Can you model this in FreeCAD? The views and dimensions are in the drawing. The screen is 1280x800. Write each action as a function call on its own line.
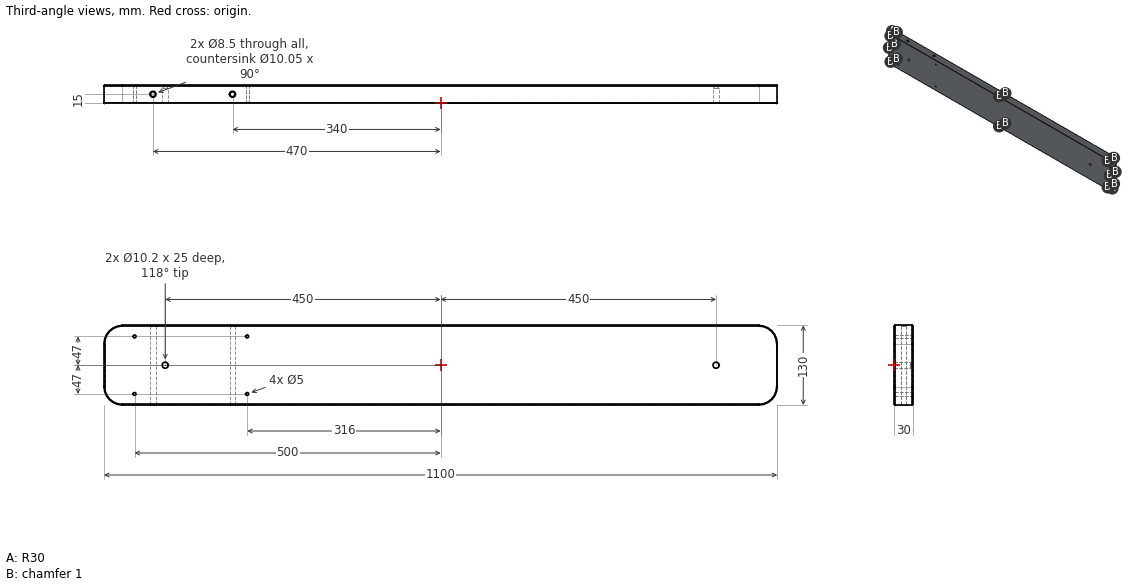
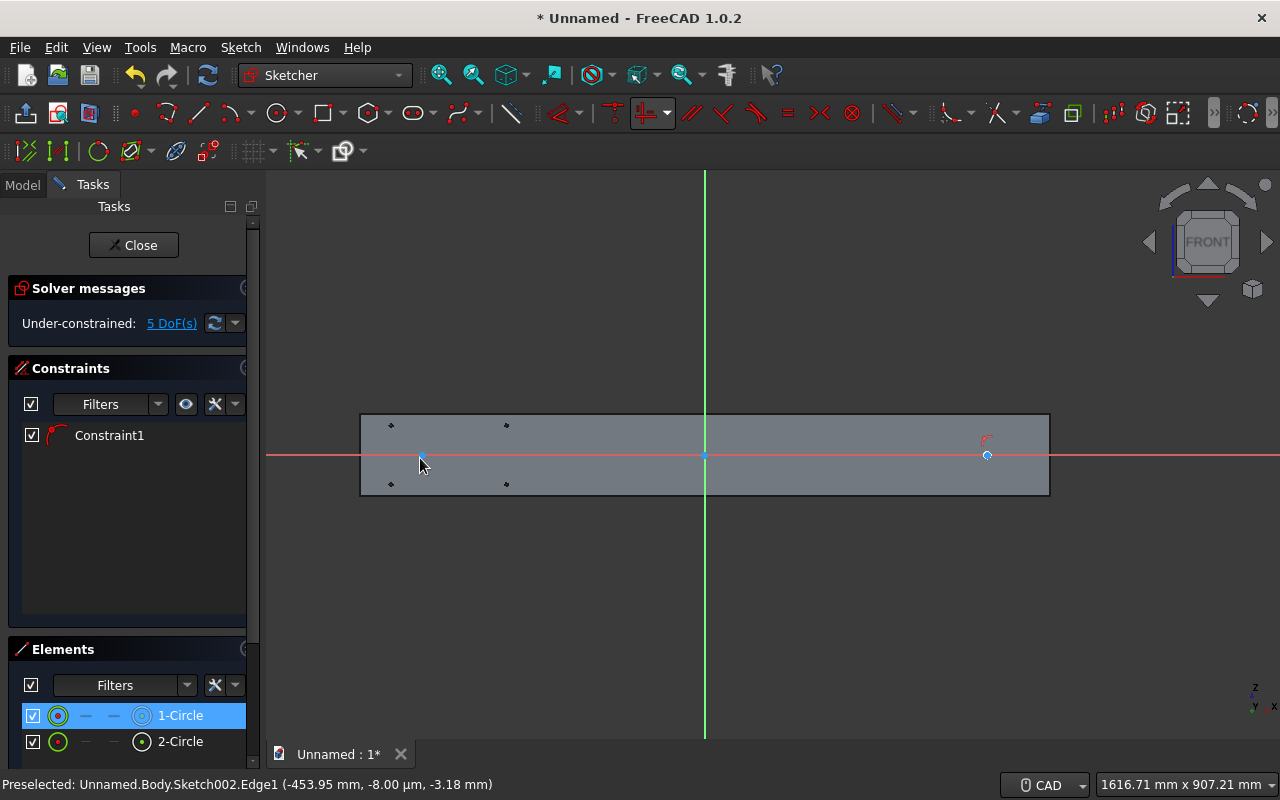
scroll(990, 453, up, 9)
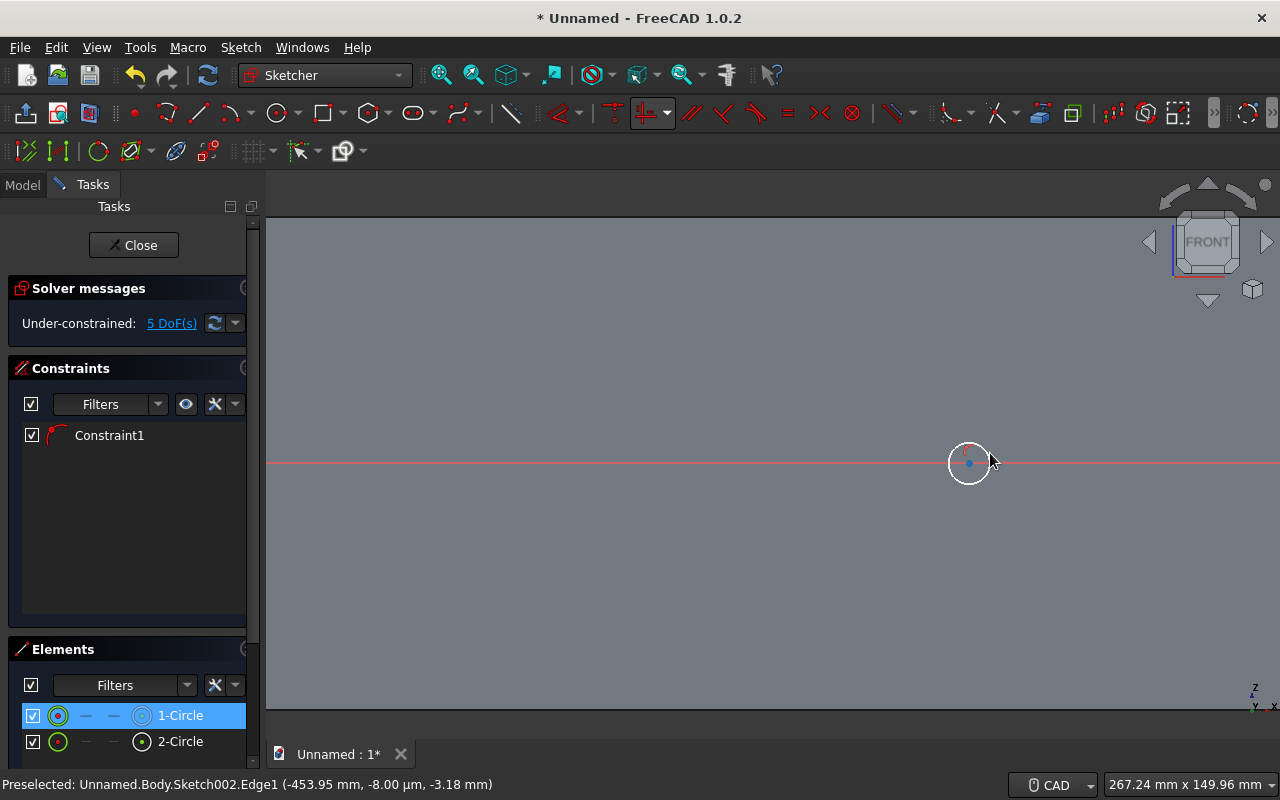
click(984, 449)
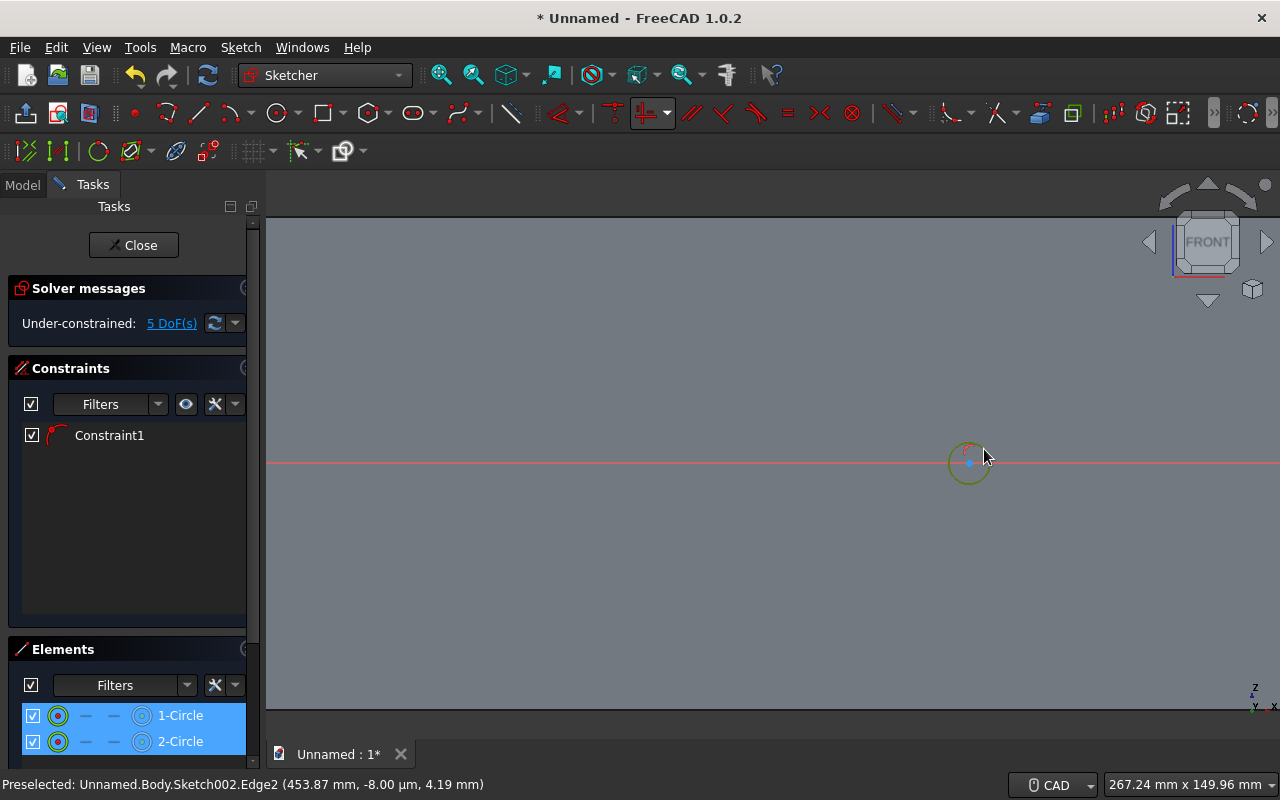
click(788, 114)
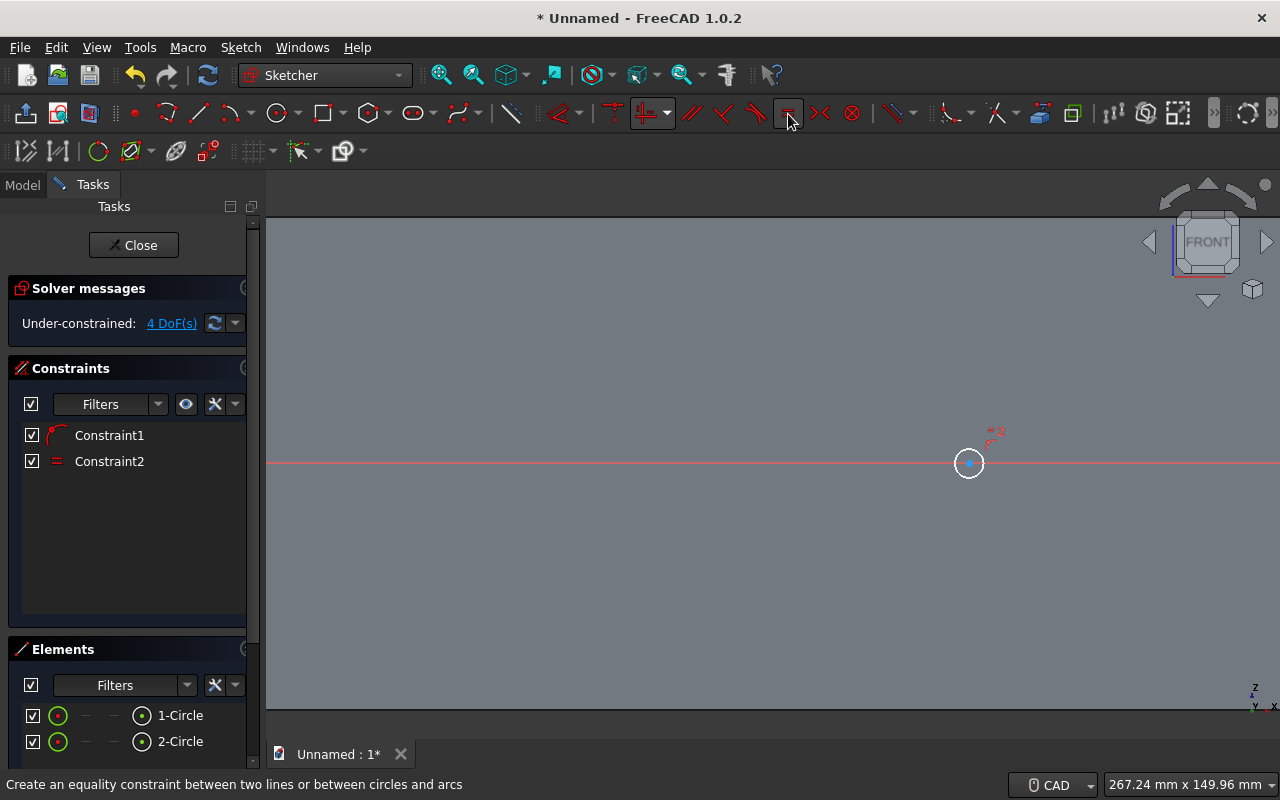
scroll(991, 453, down, 9)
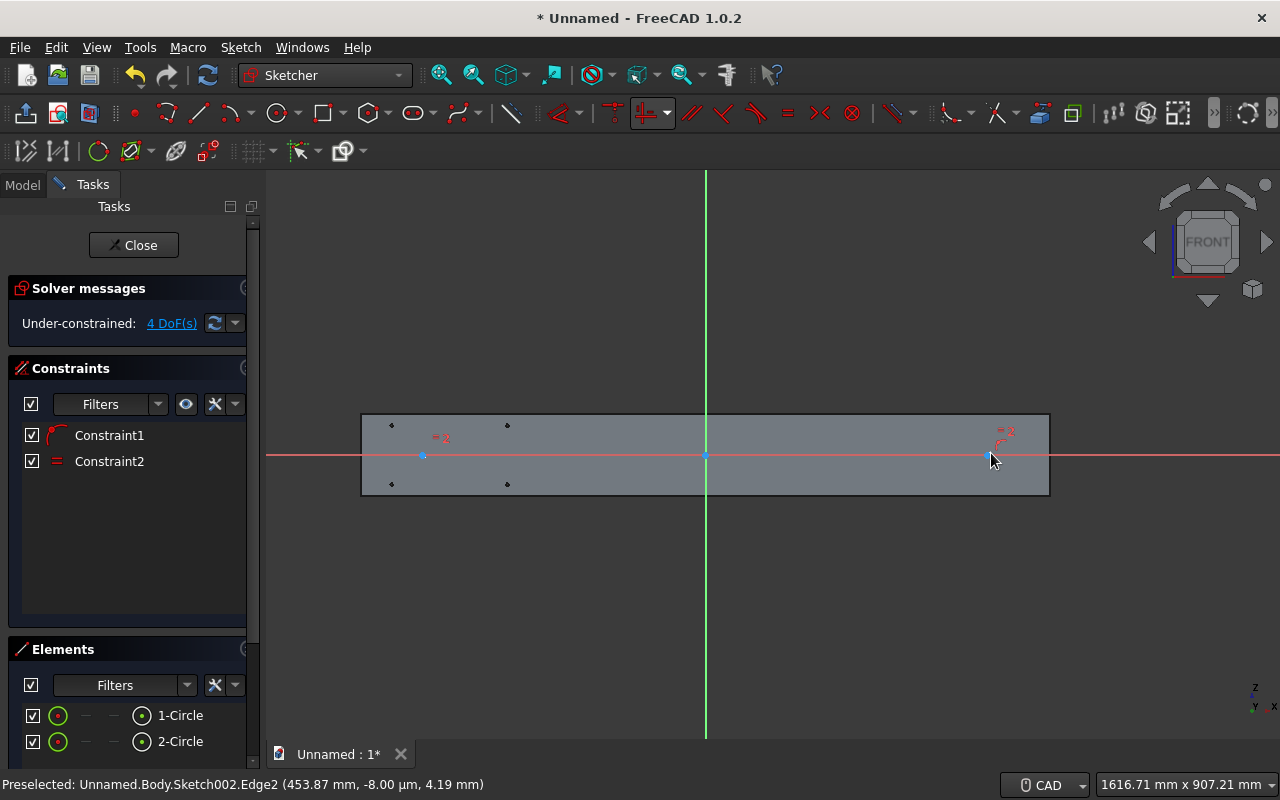
click(423, 456)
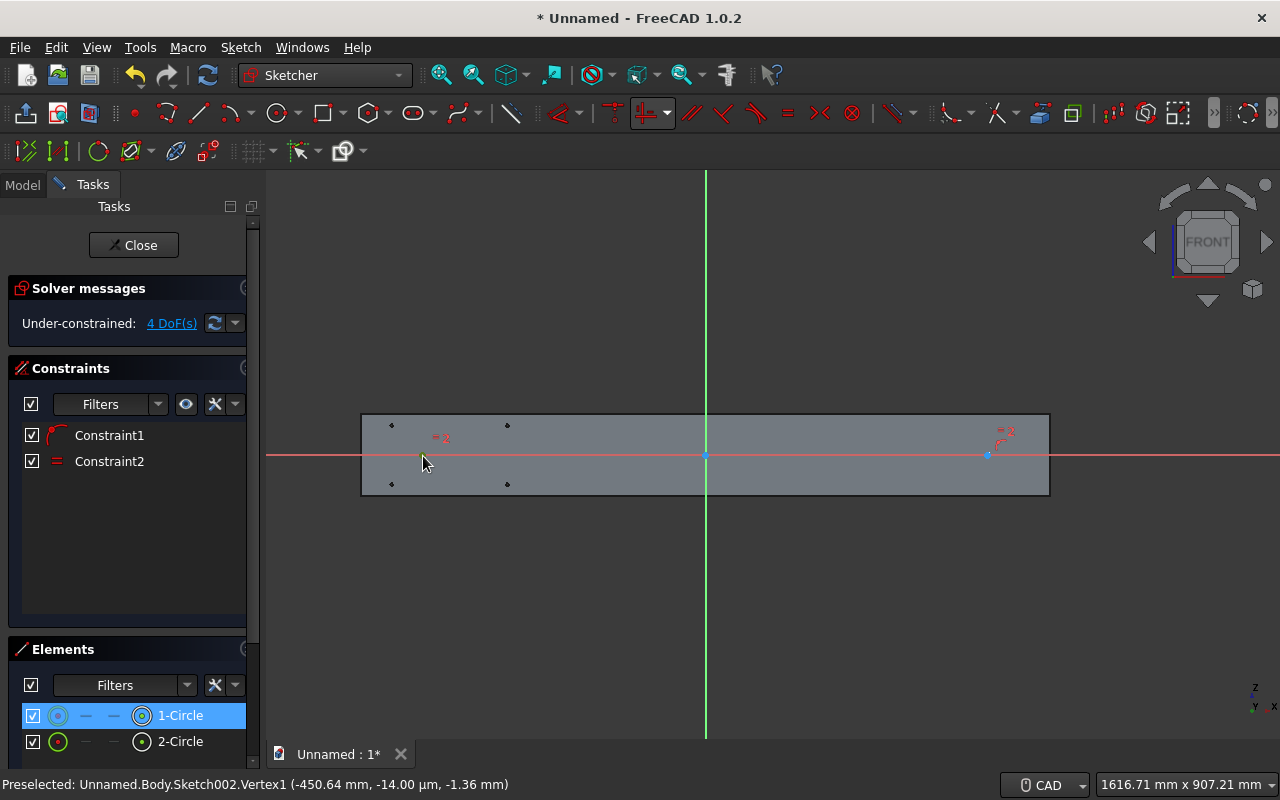
click(353, 455)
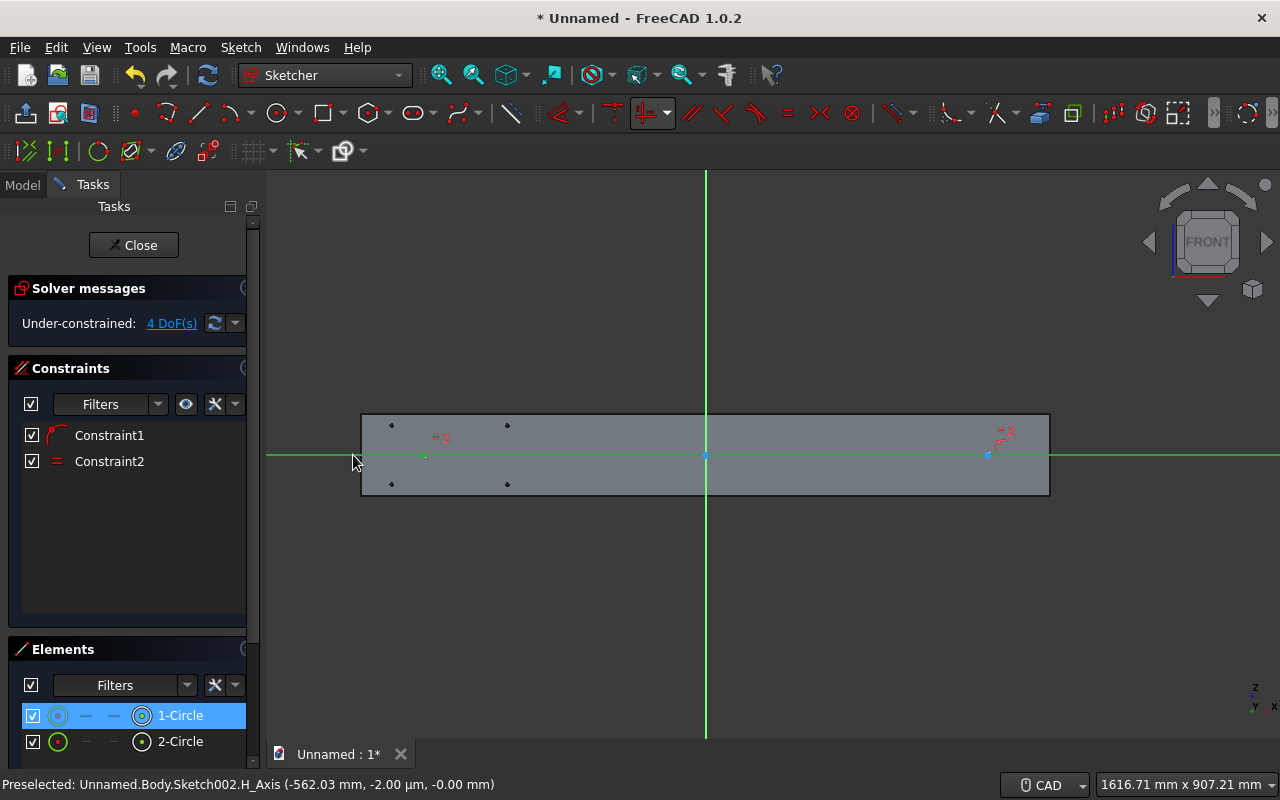
click(614, 114)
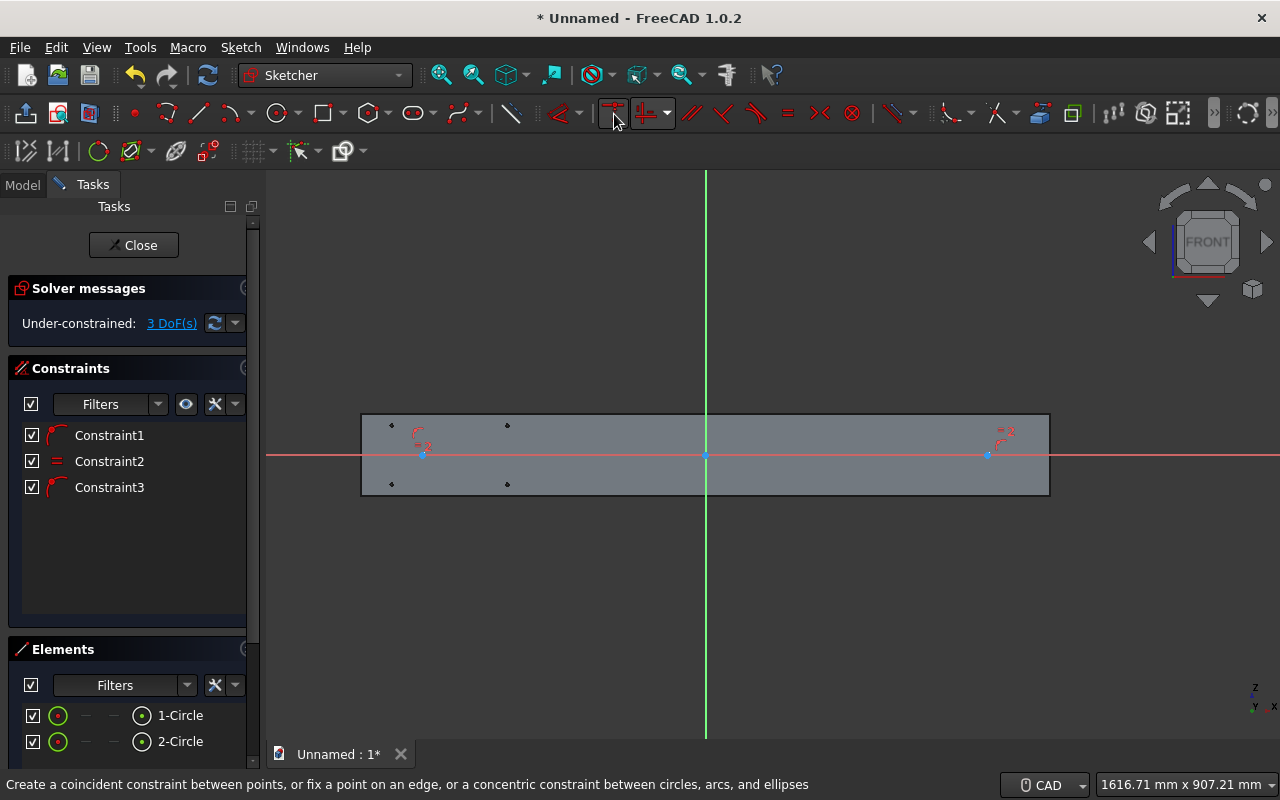
click(558, 114)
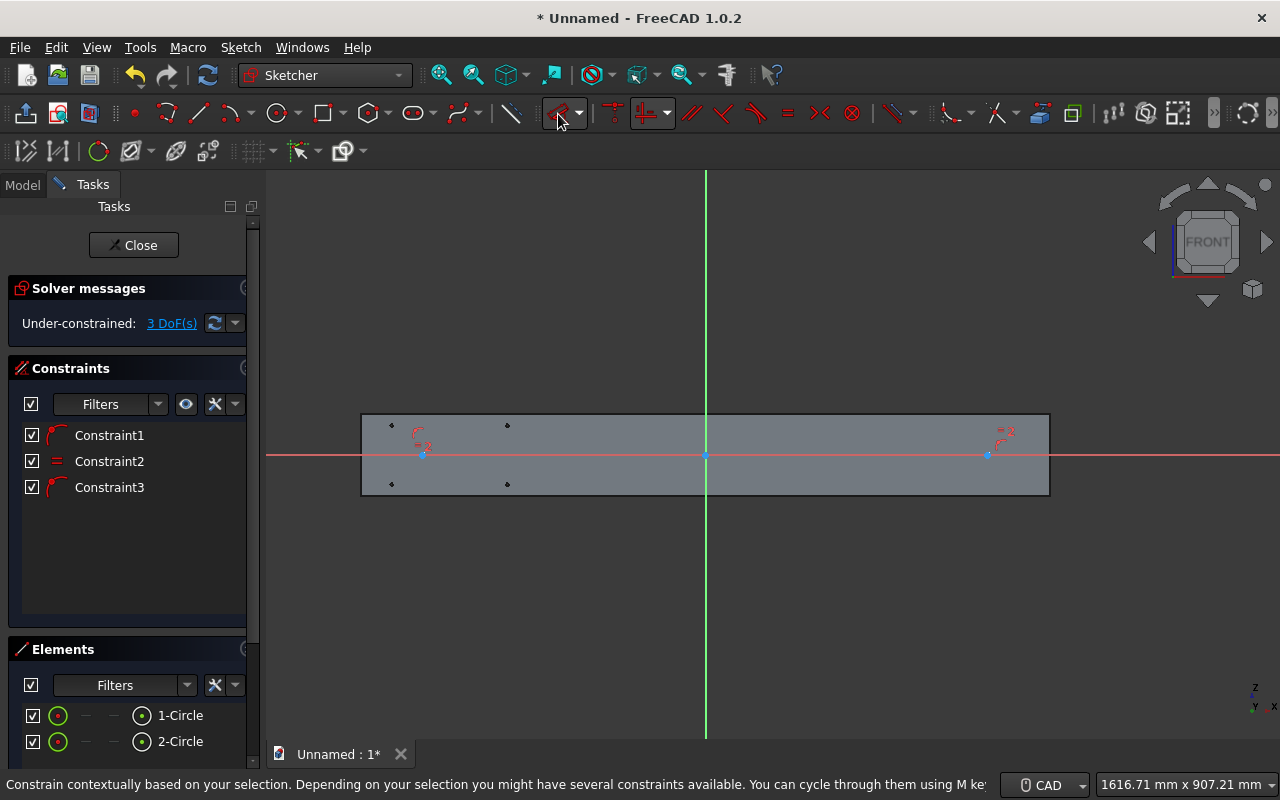
scroll(423, 453, up, 10)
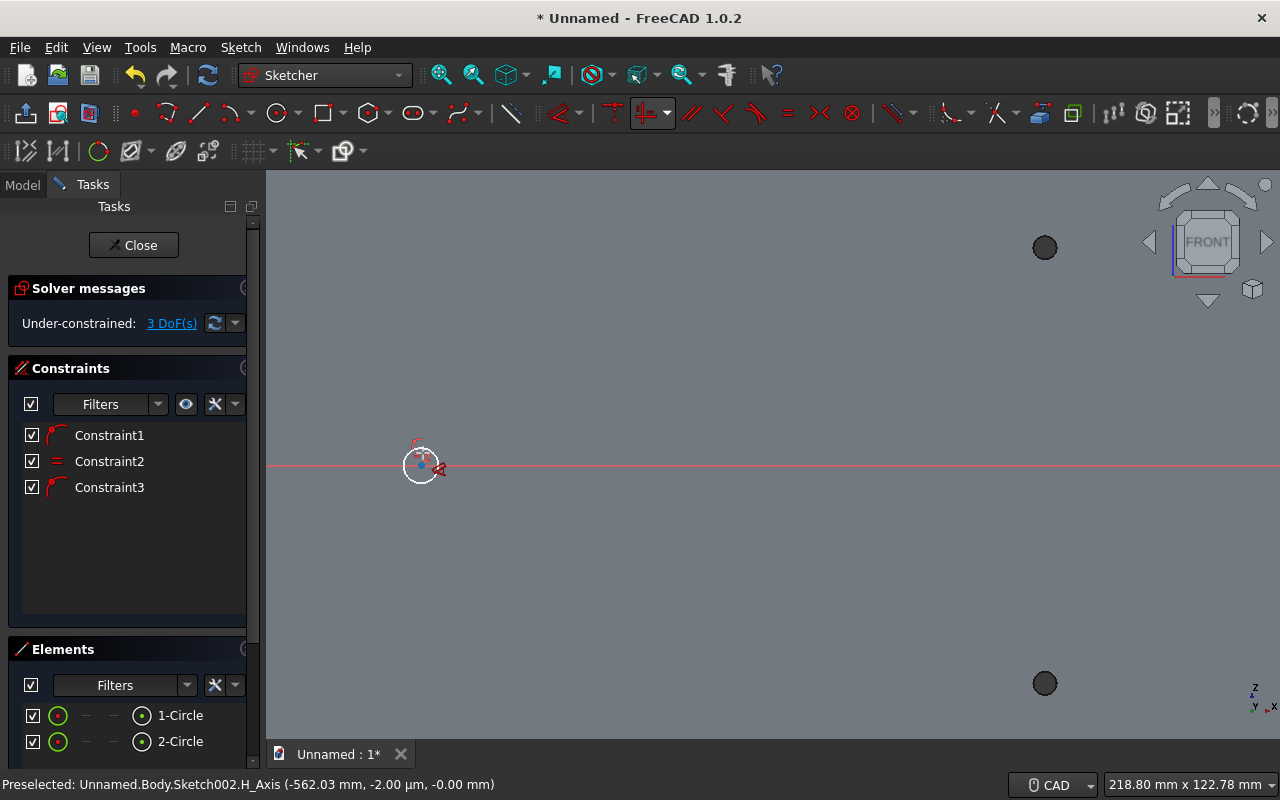
click(422, 448)
click(424, 416)